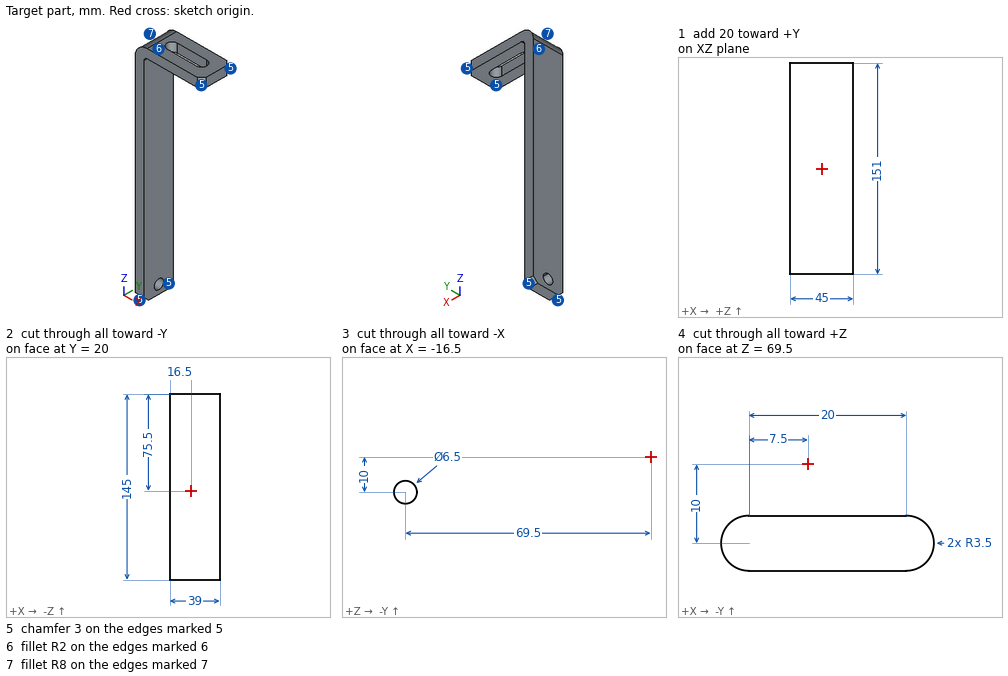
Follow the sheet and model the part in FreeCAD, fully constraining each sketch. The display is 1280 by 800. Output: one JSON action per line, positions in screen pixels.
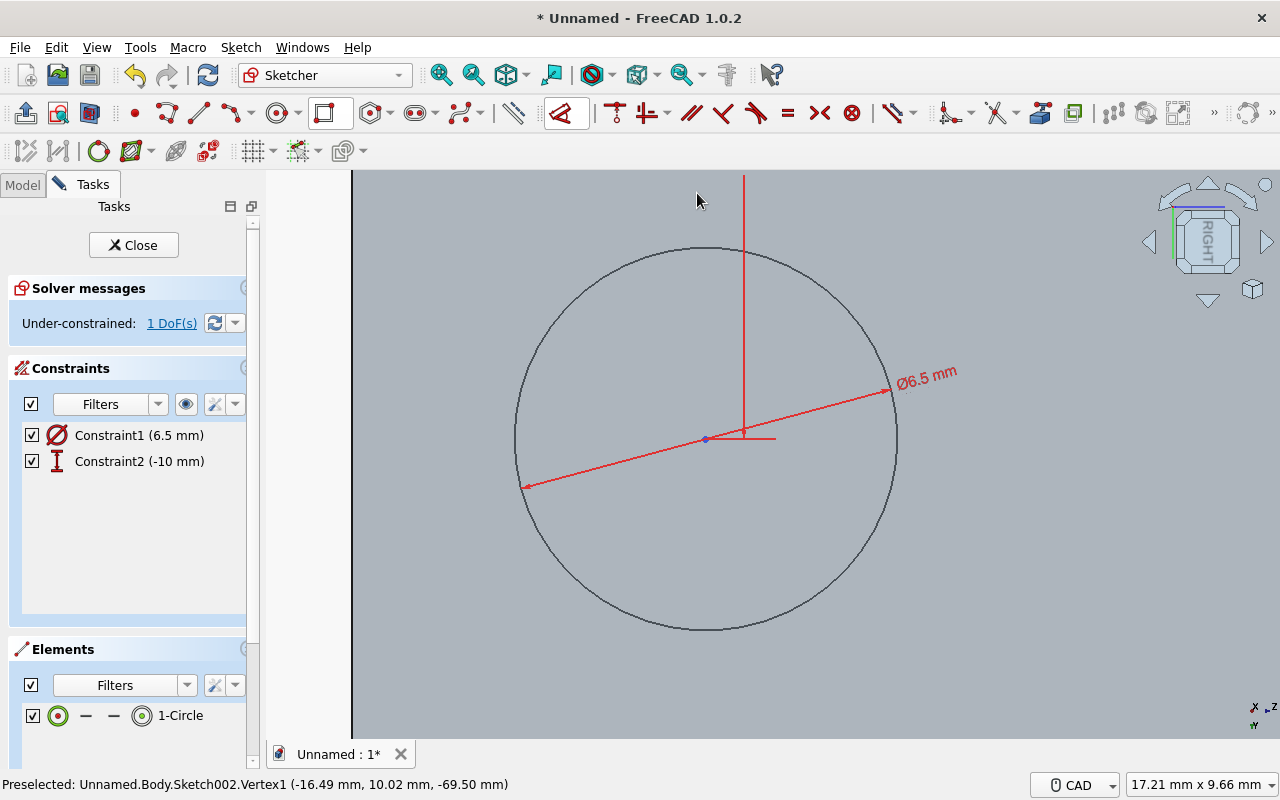
{"action": "left_click", "coordinate": [706, 439]}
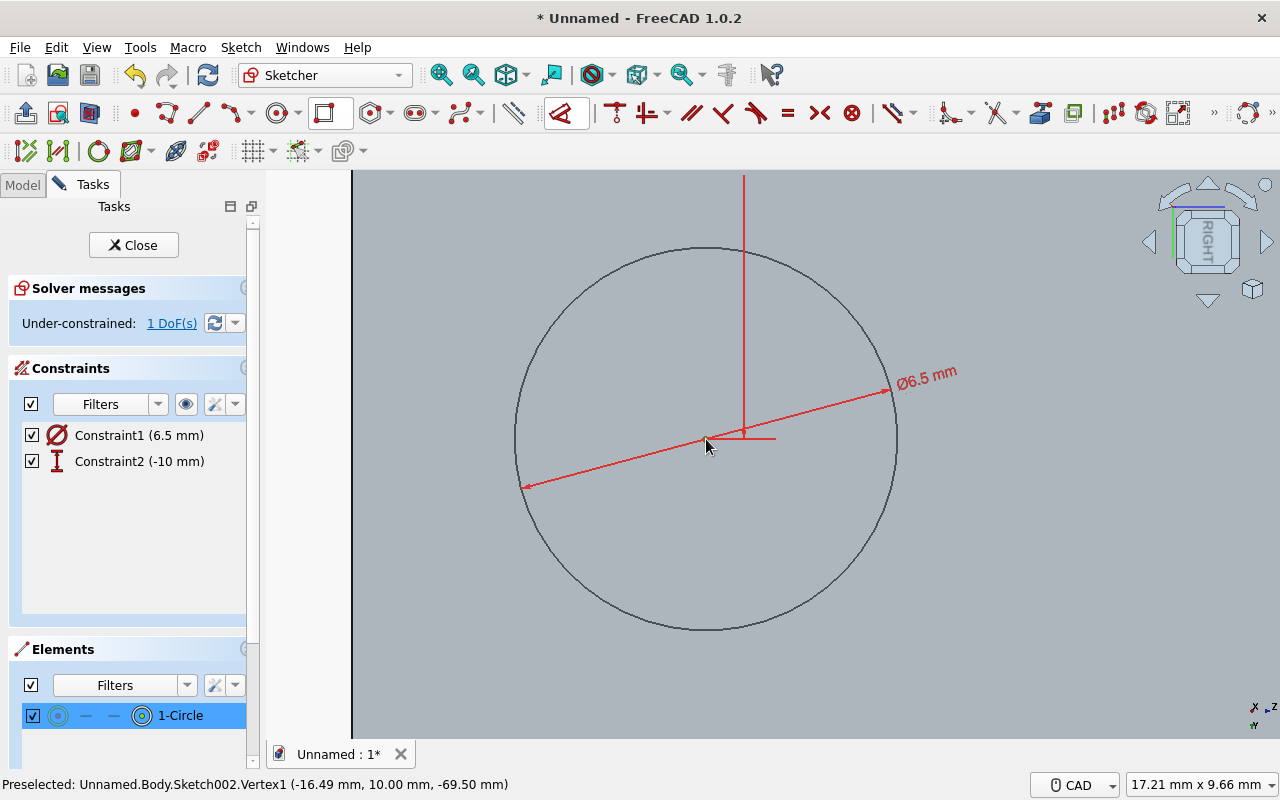
{"action": "left_click", "coordinate": [584, 114]}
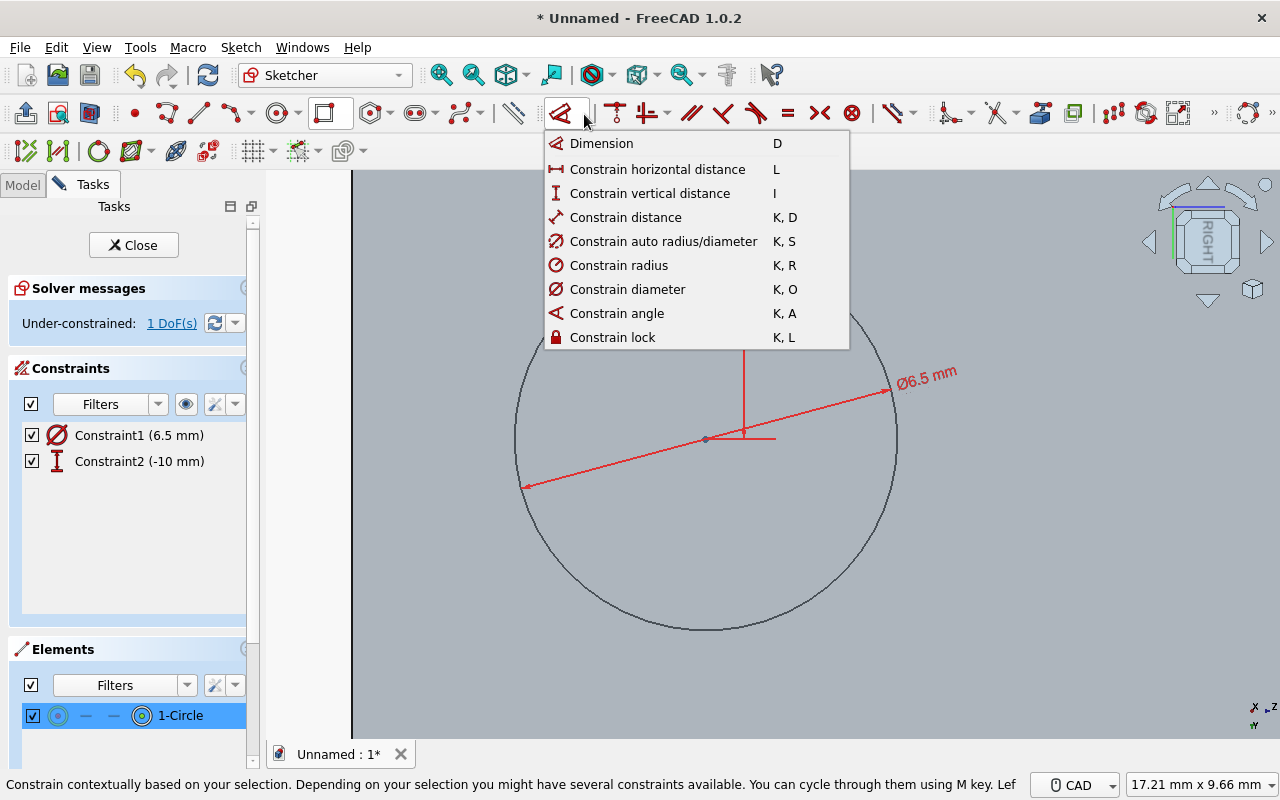
{"action": "left_click", "coordinate": [697, 169]}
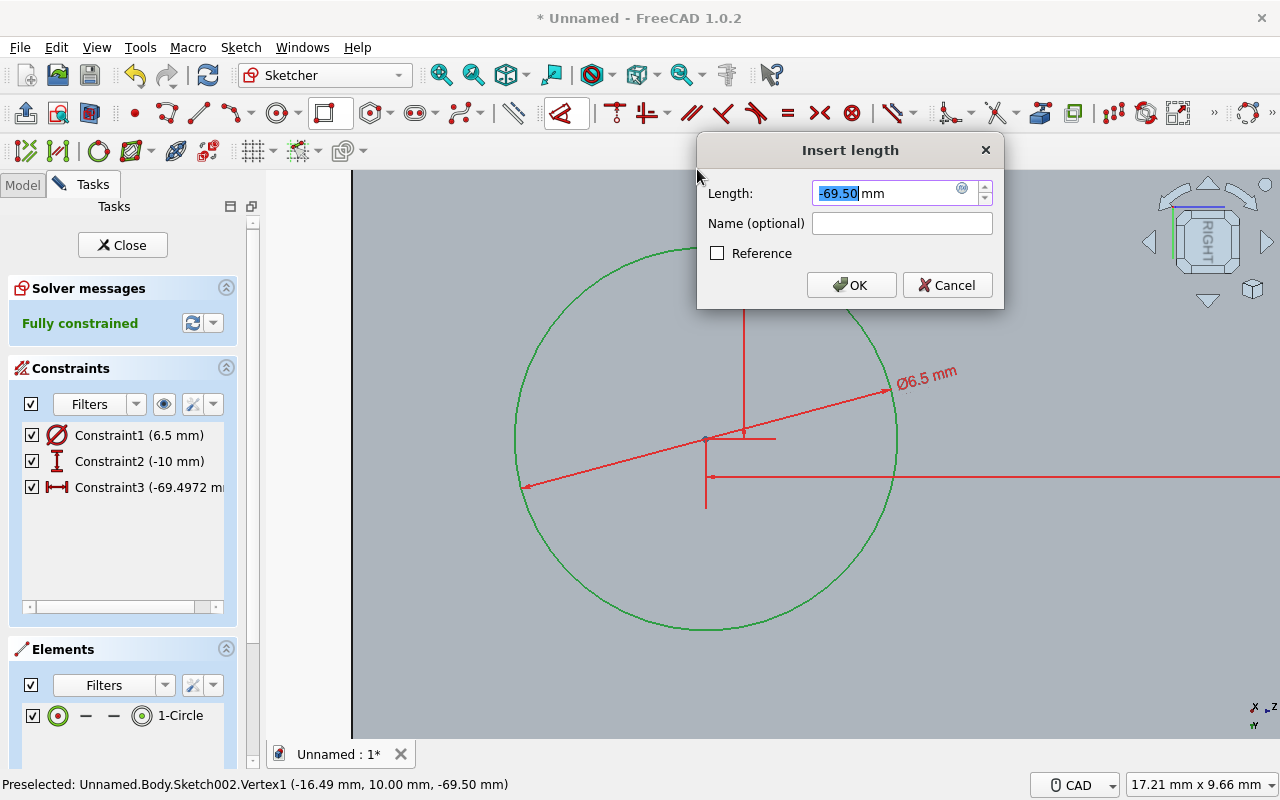
{"action": "type", "text": "-69.5"}
{"action": "key", "text": "Return"}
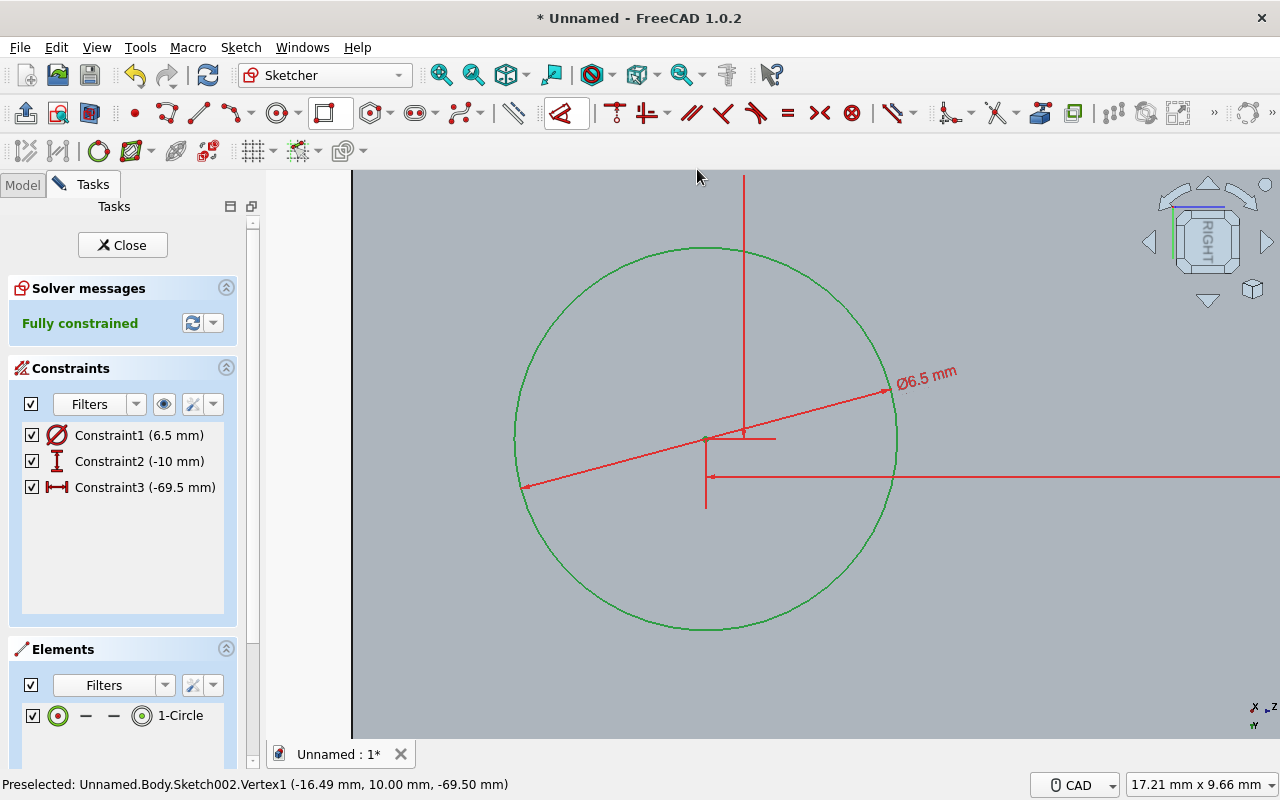
{"action": "left_click", "coordinate": [123, 245]}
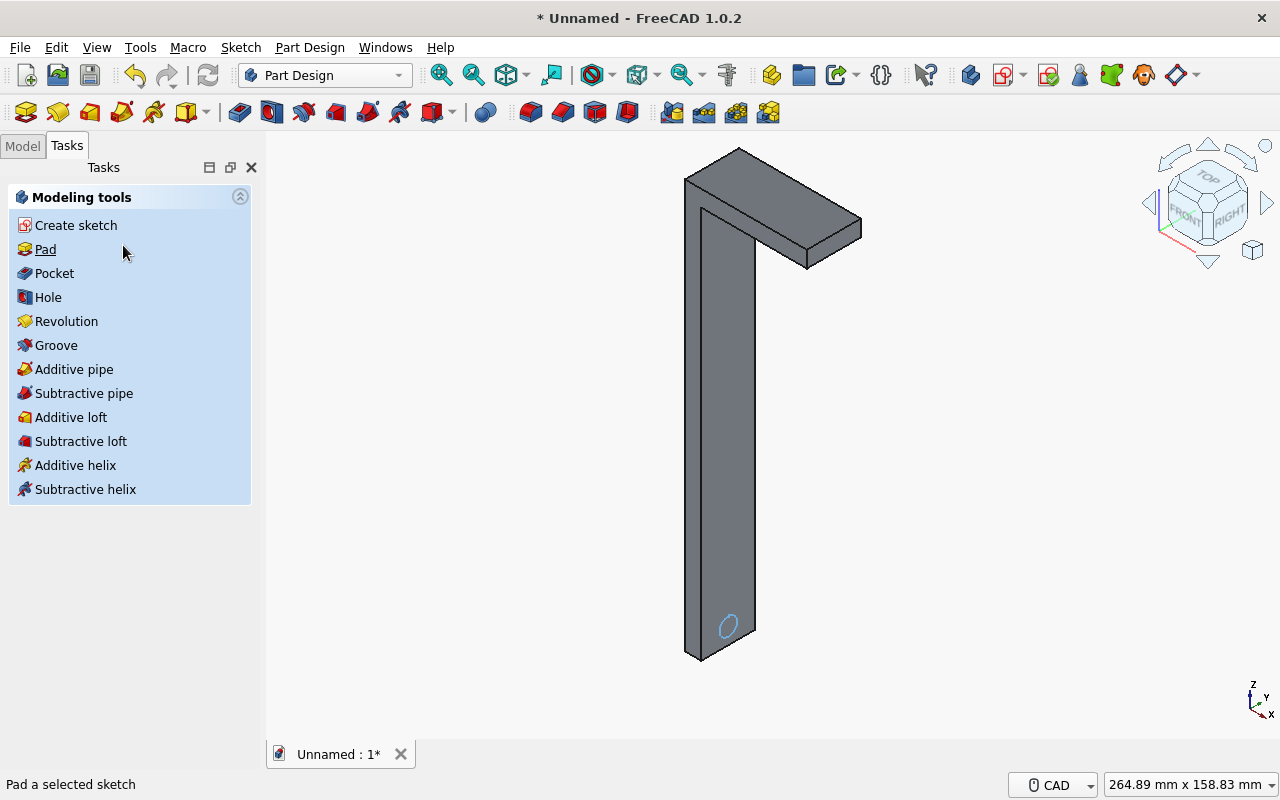
{"action": "left_click", "coordinate": [240, 112]}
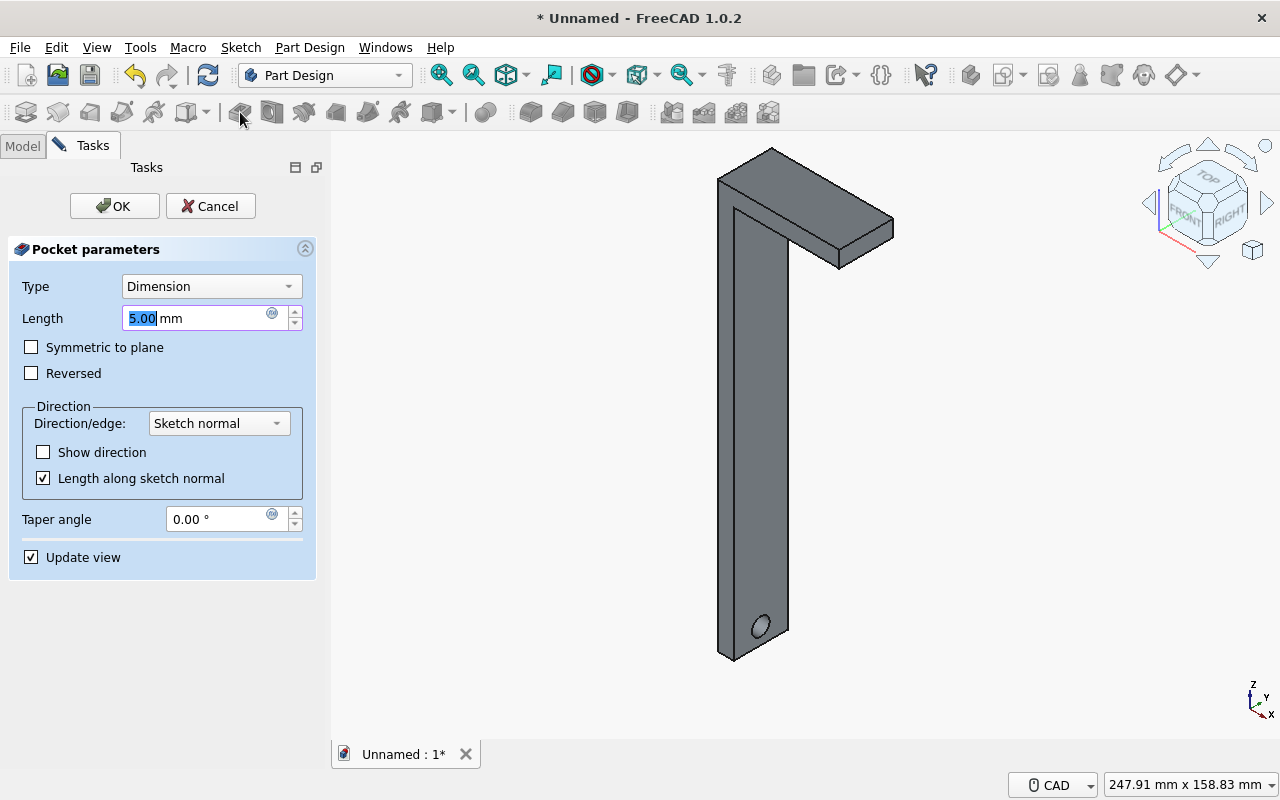
{"action": "left_click", "coordinate": [212, 286]}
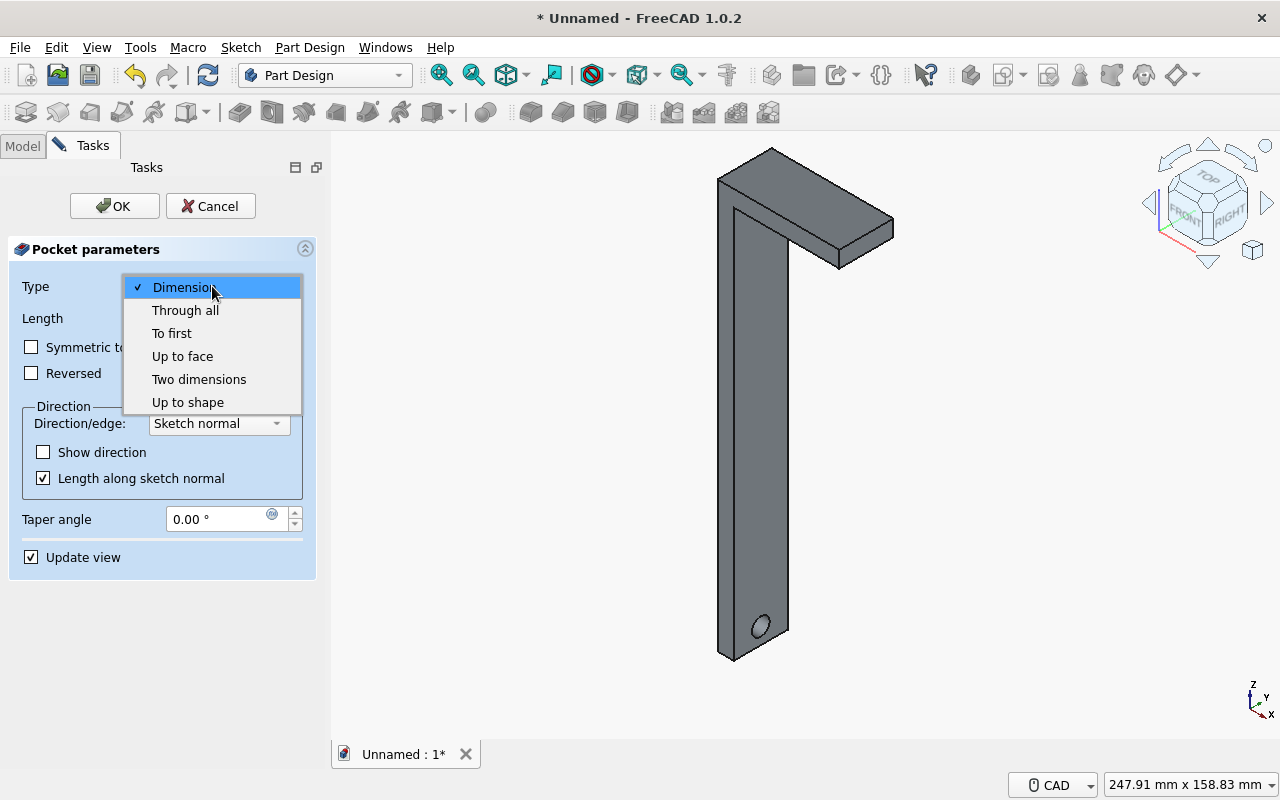
{"action": "left_click", "coordinate": [212, 310]}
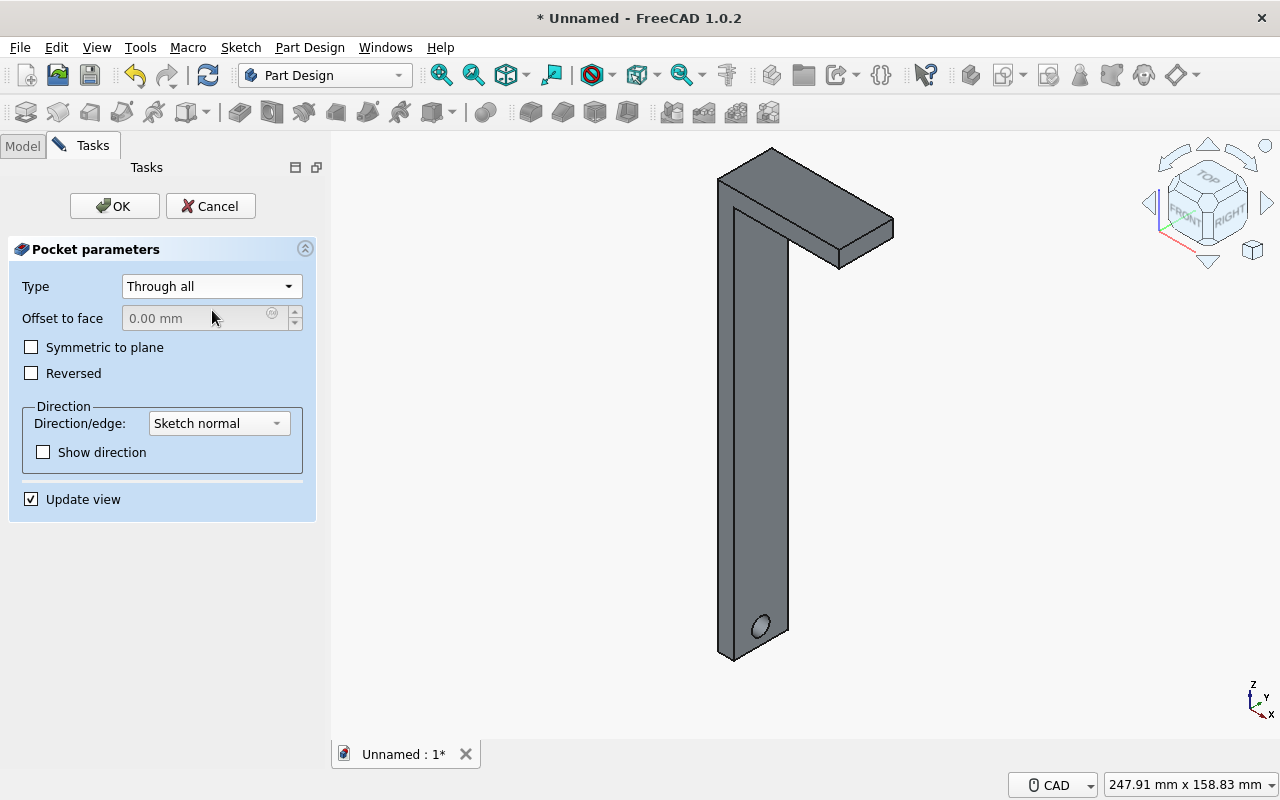
{"action": "left_click", "coordinate": [115, 206]}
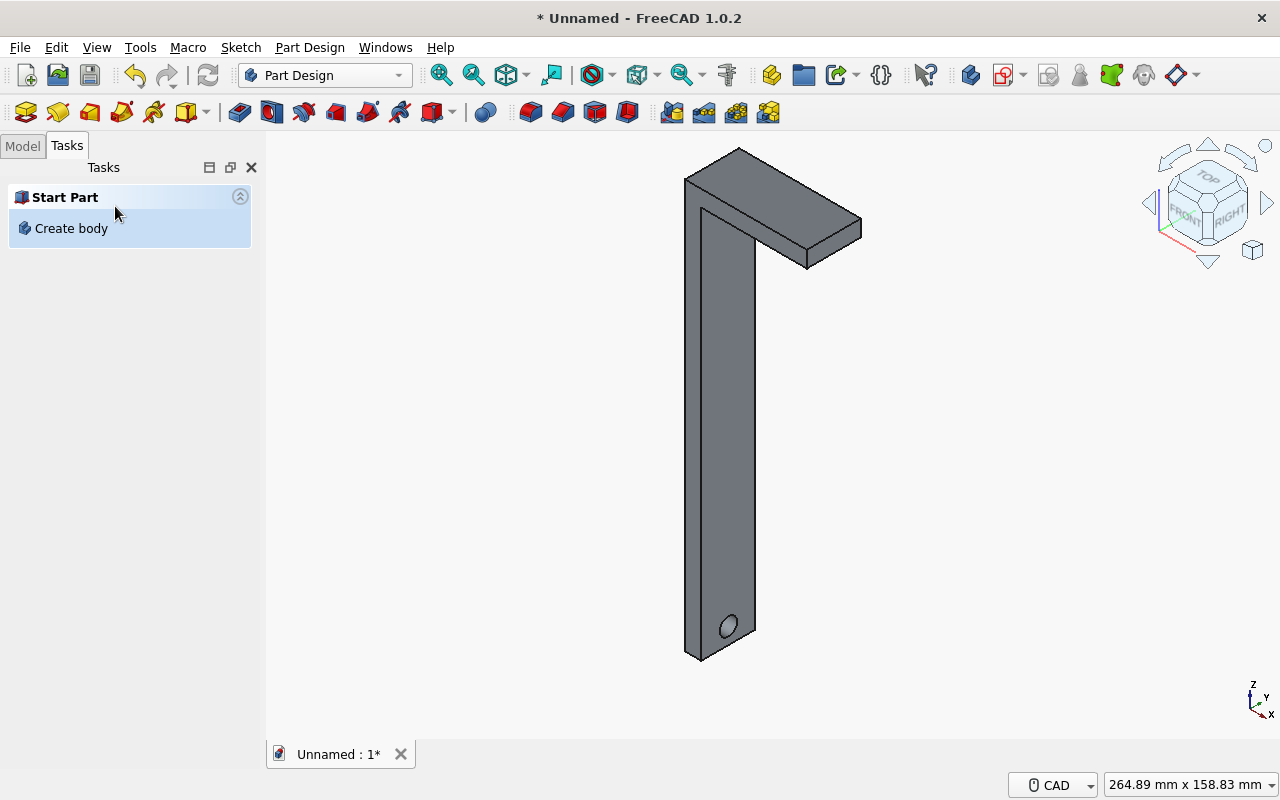
{"action": "key", "text": "5"}